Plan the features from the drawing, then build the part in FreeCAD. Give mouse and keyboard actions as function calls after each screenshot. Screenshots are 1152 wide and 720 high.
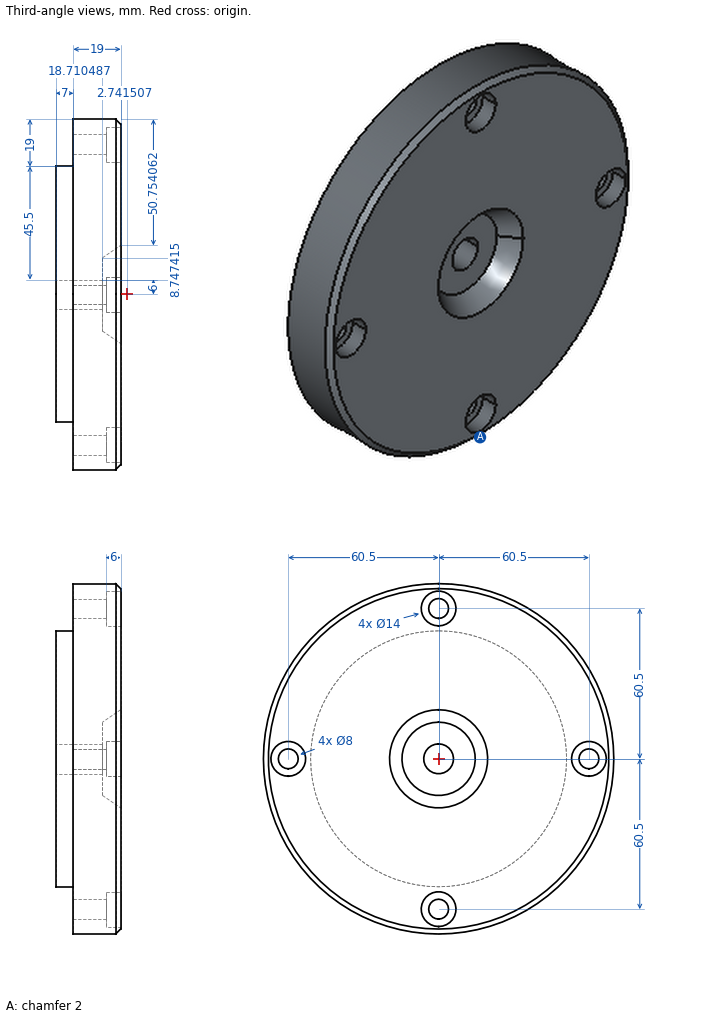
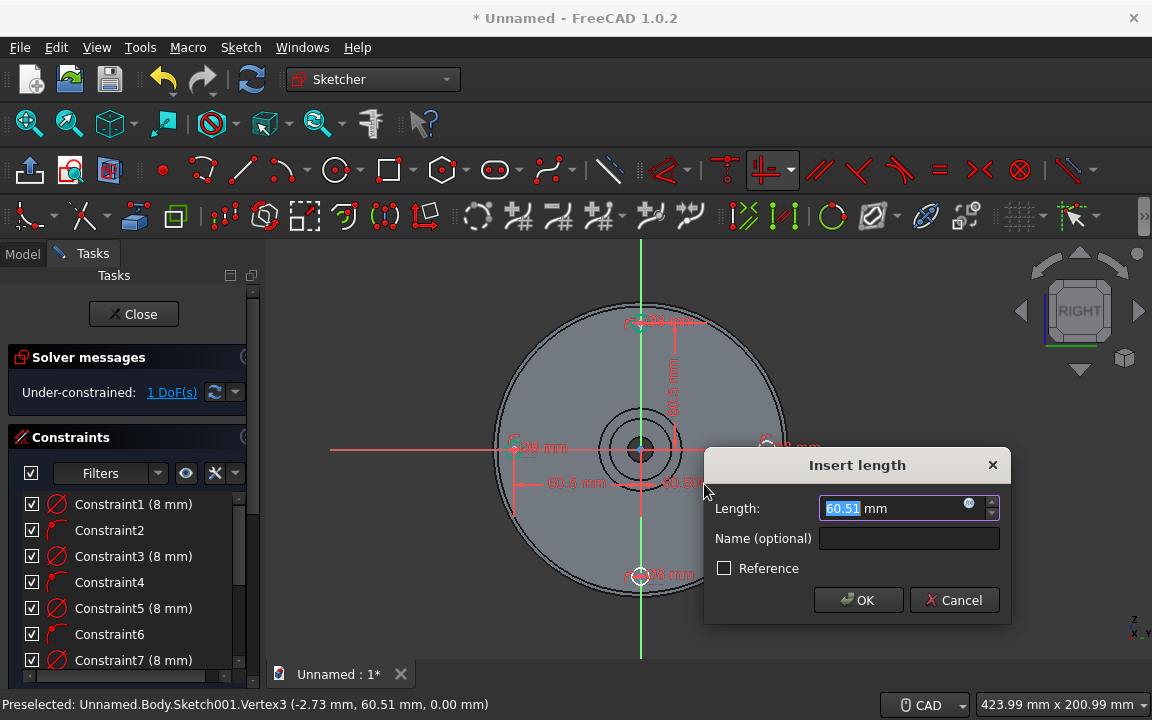
text(60.5)
key(Return)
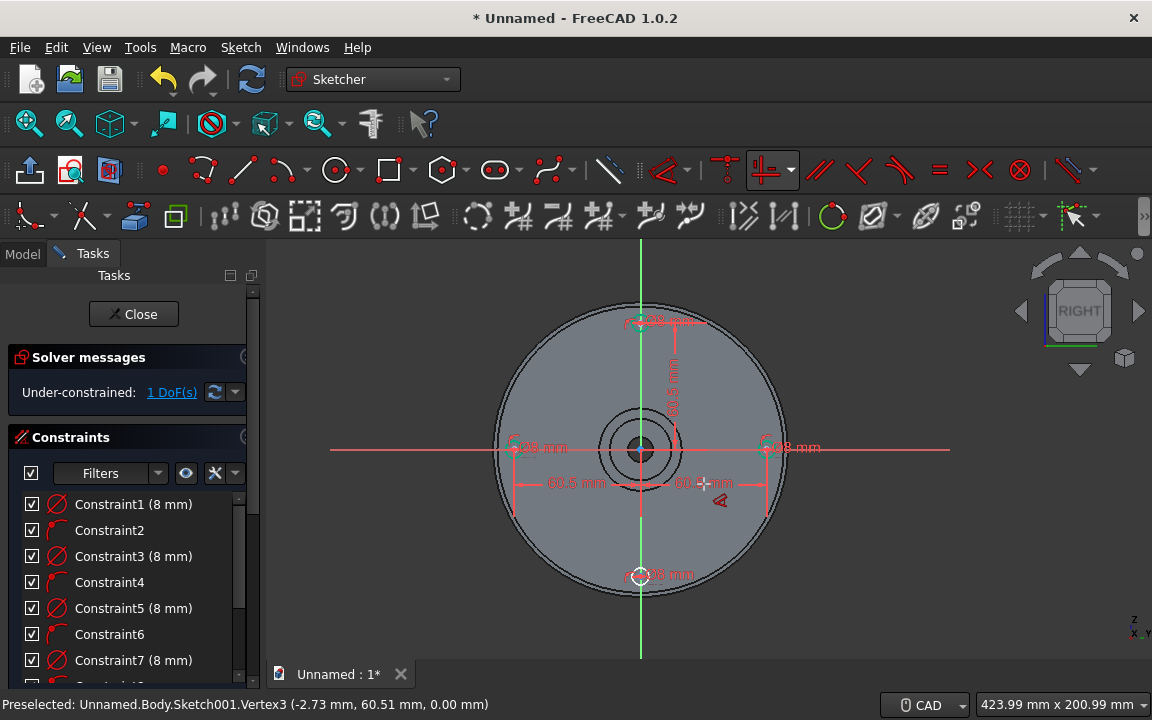
click(641, 577)
click(675, 513)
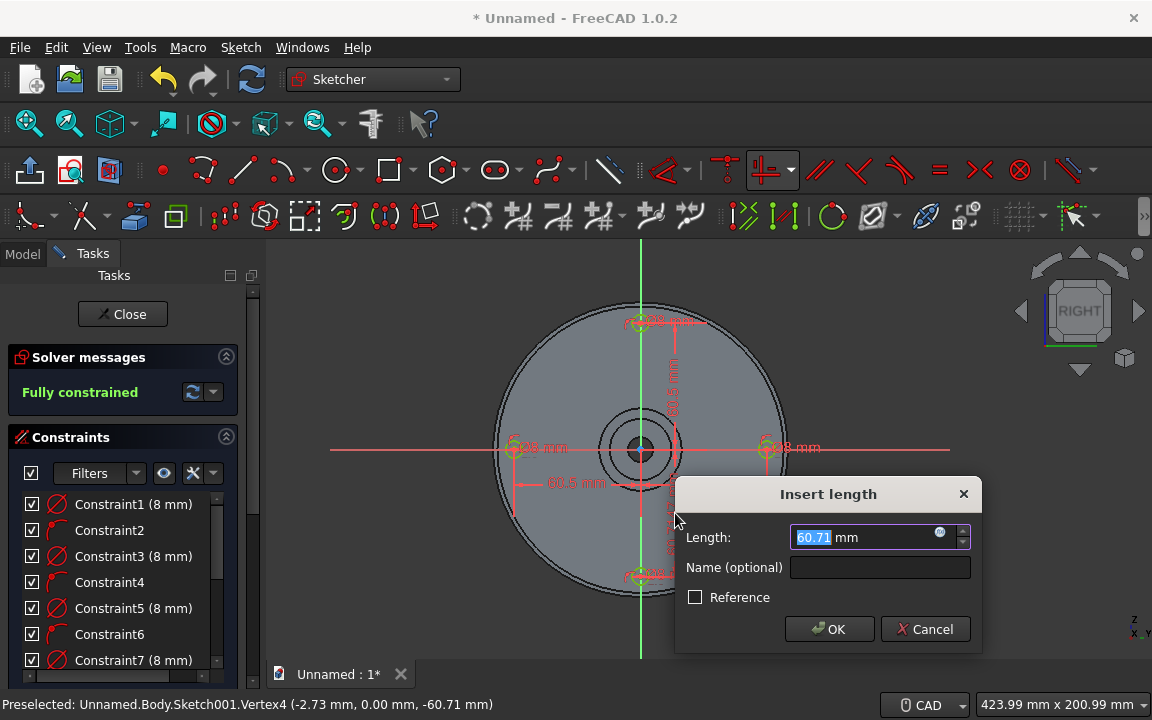
text(60.5)
key(Return)
key(Escape)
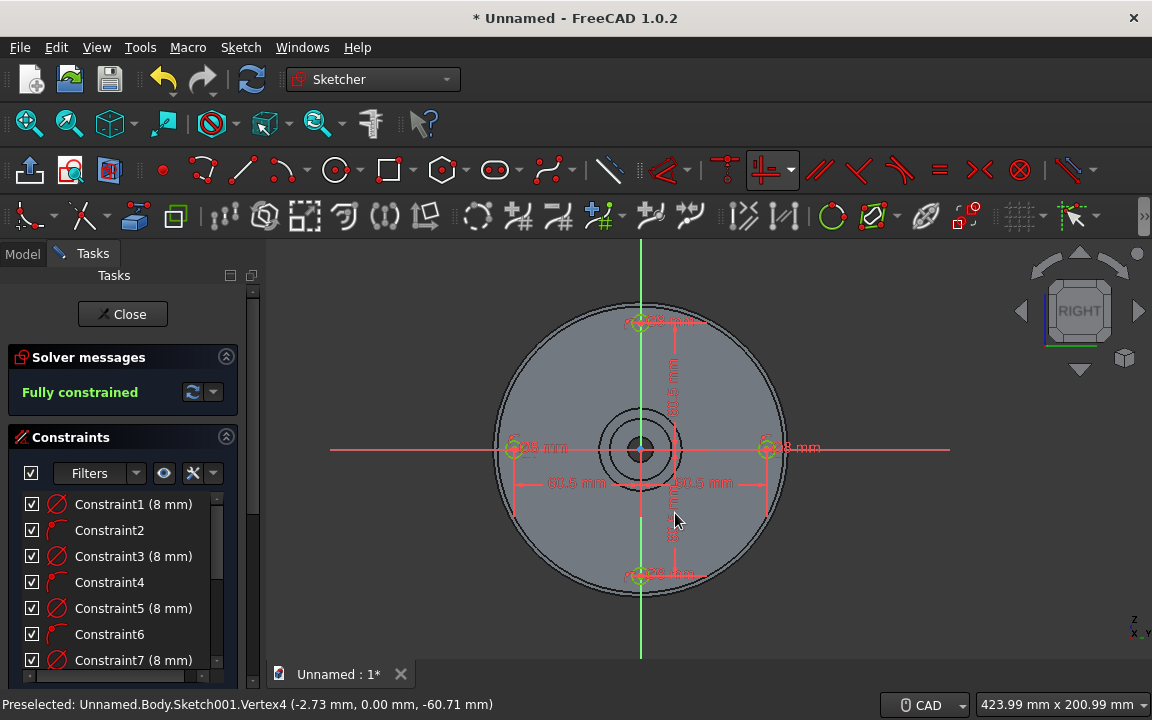
click(123, 314)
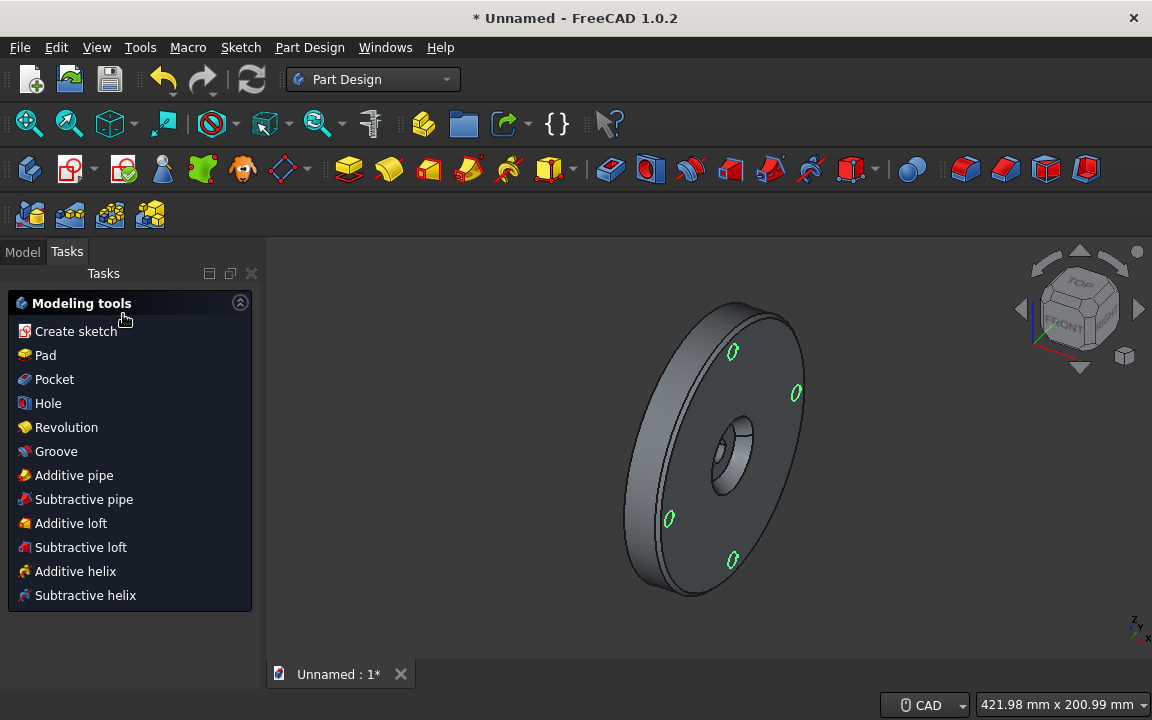
click(612, 170)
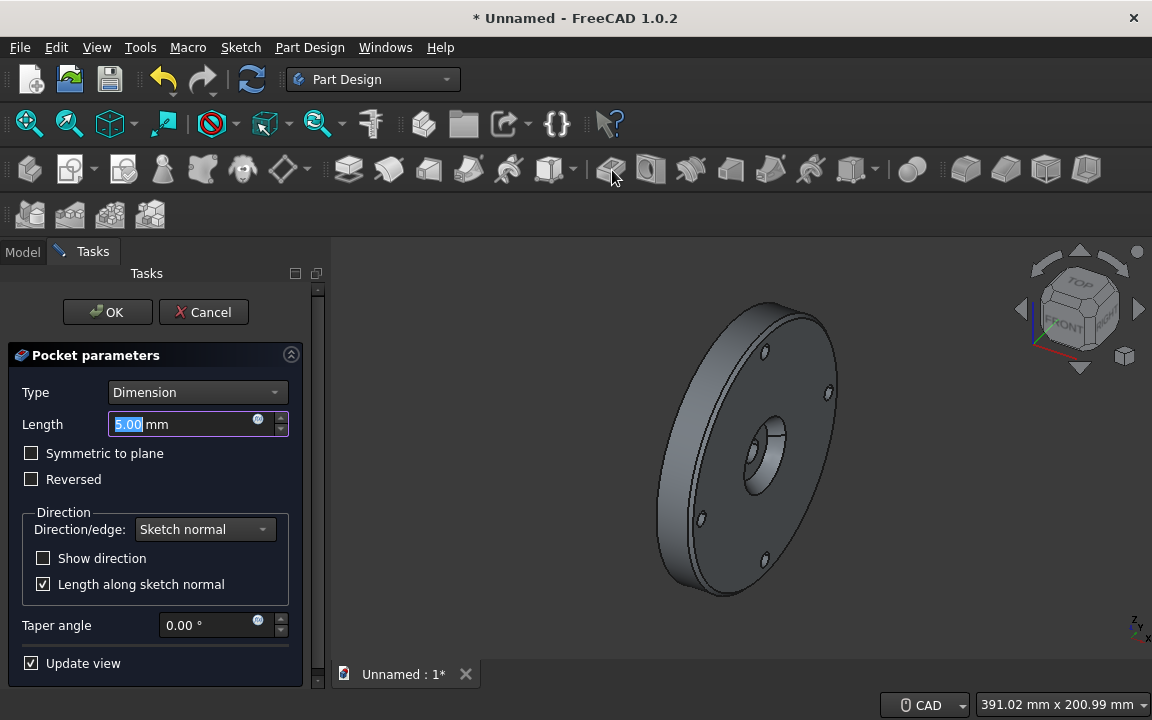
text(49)
key(Tab)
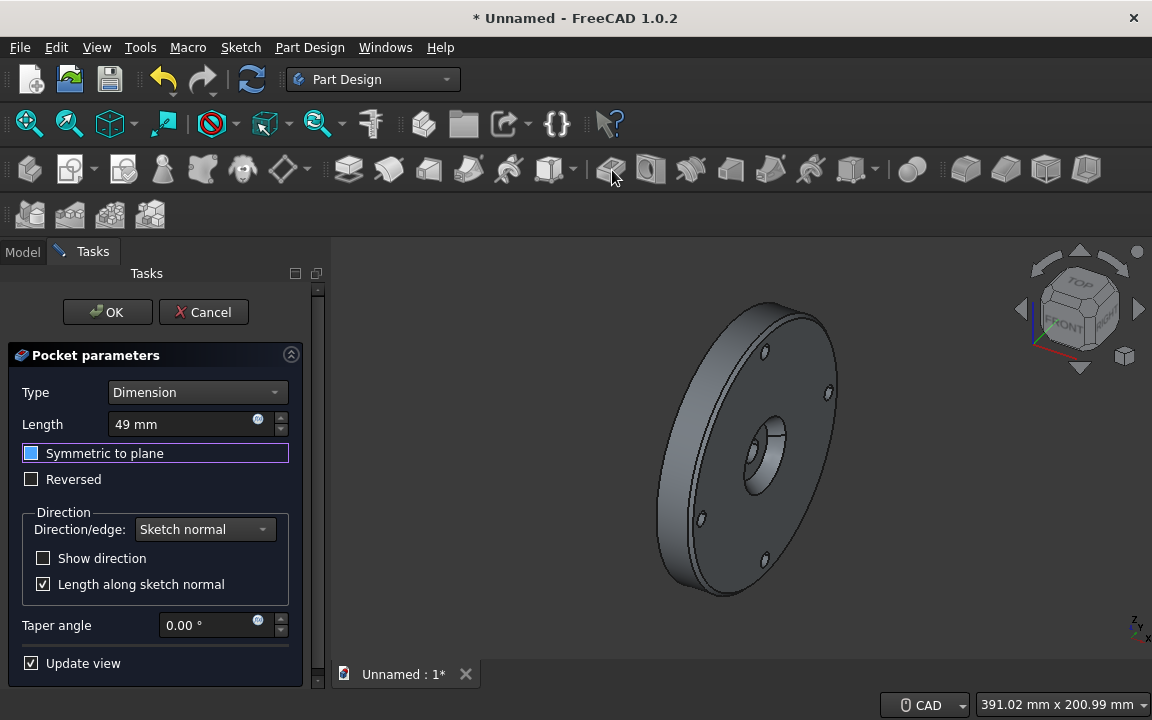
click(108, 312)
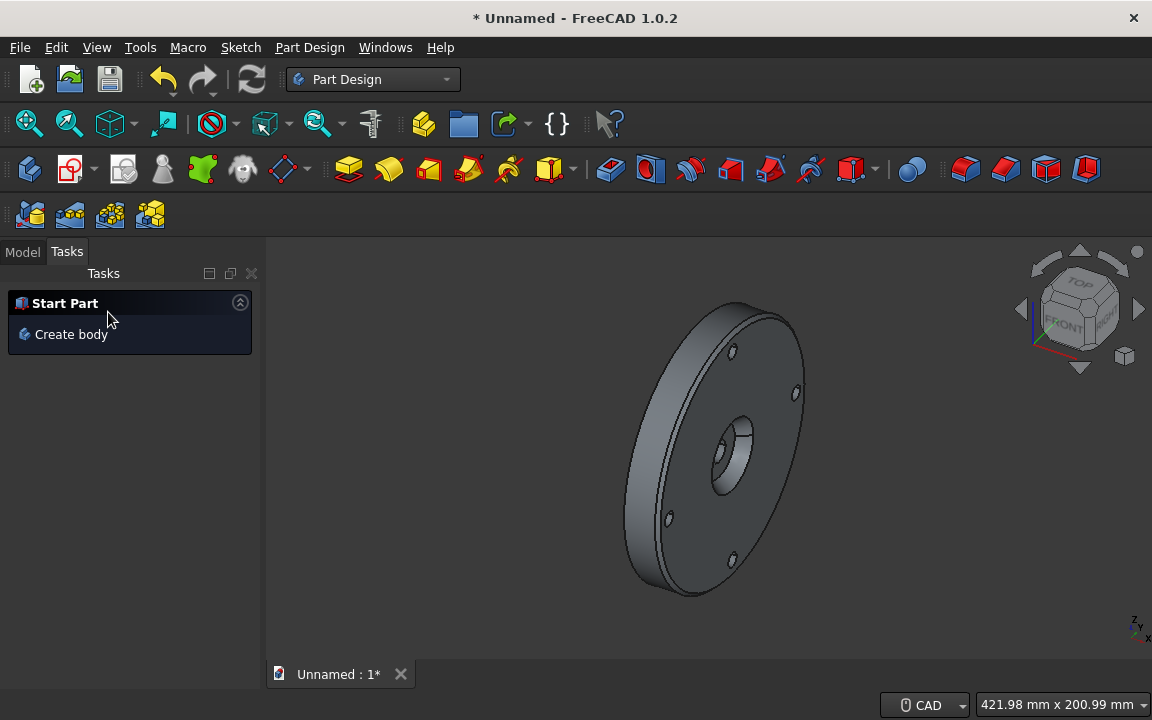
click(774, 380)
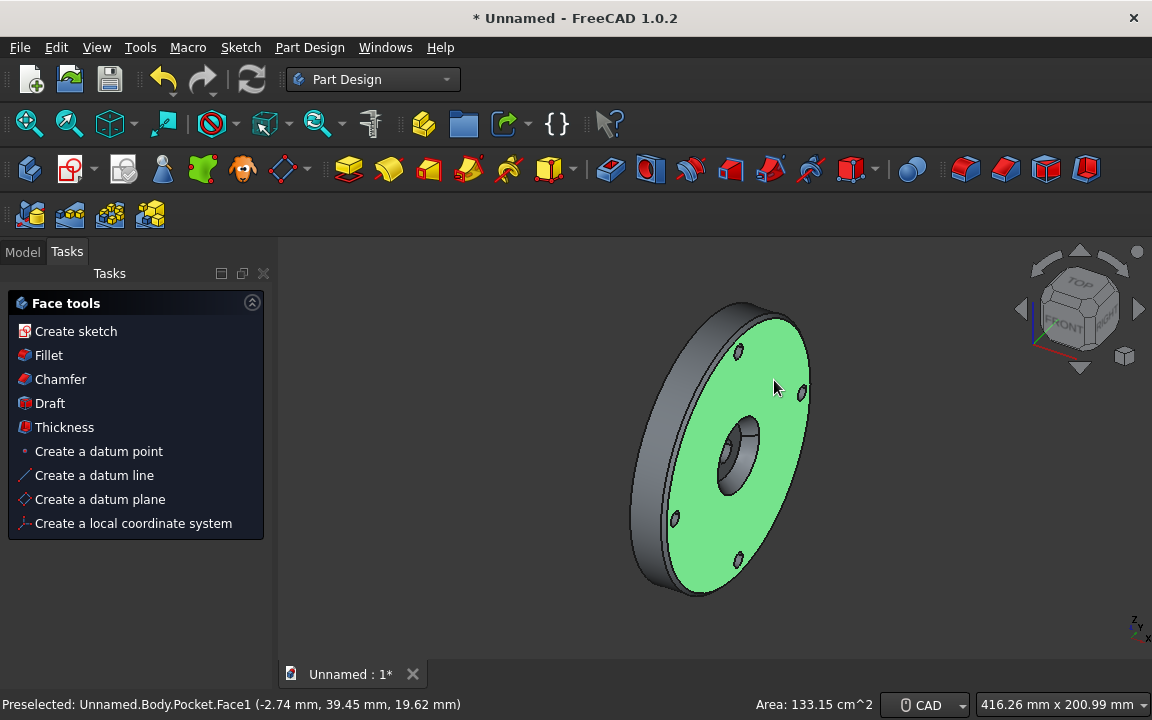
click(70, 170)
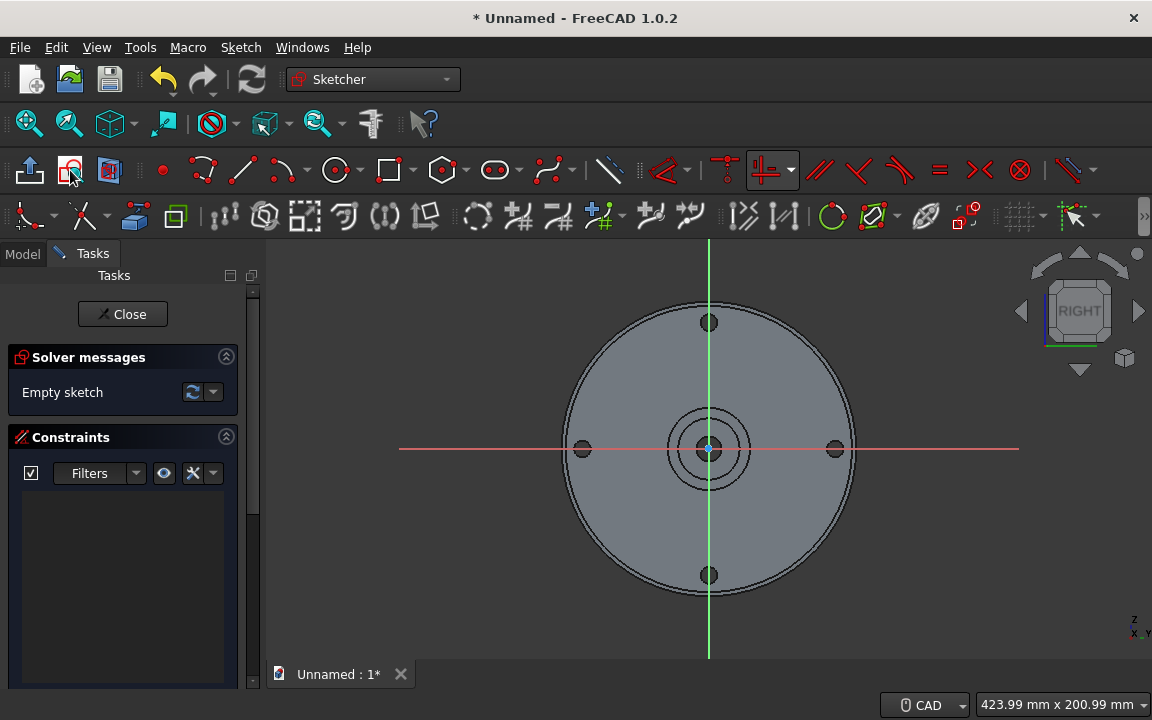
click(336, 170)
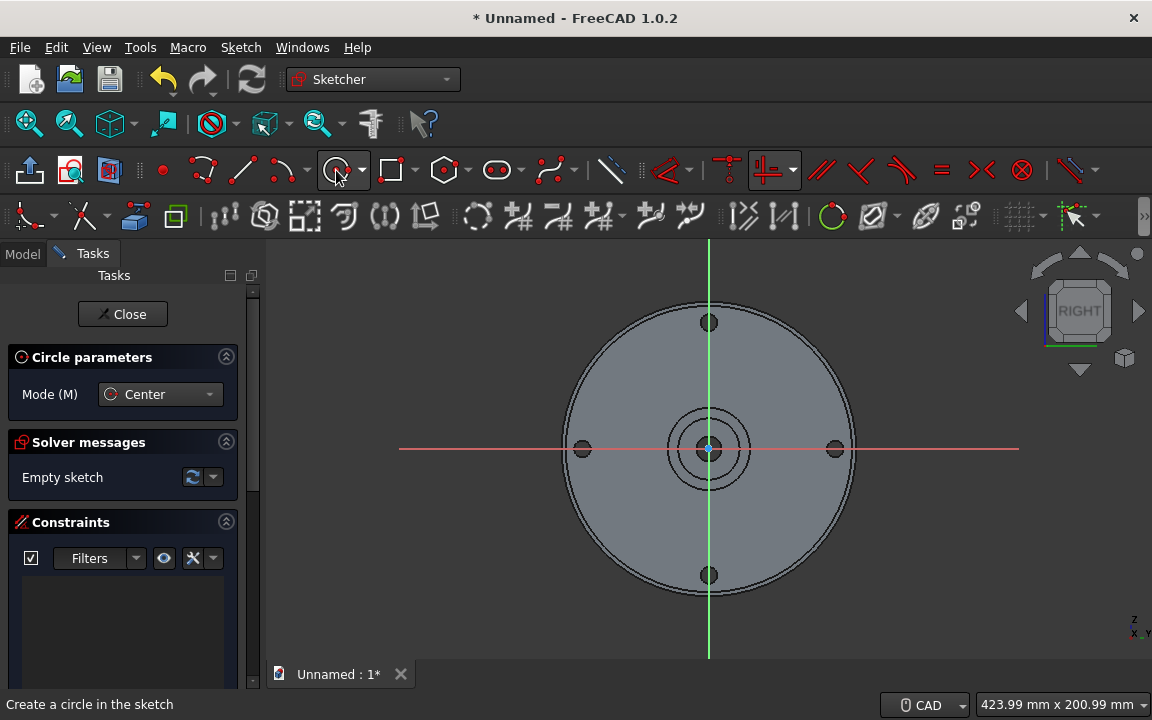
scroll(709, 323, up, 3)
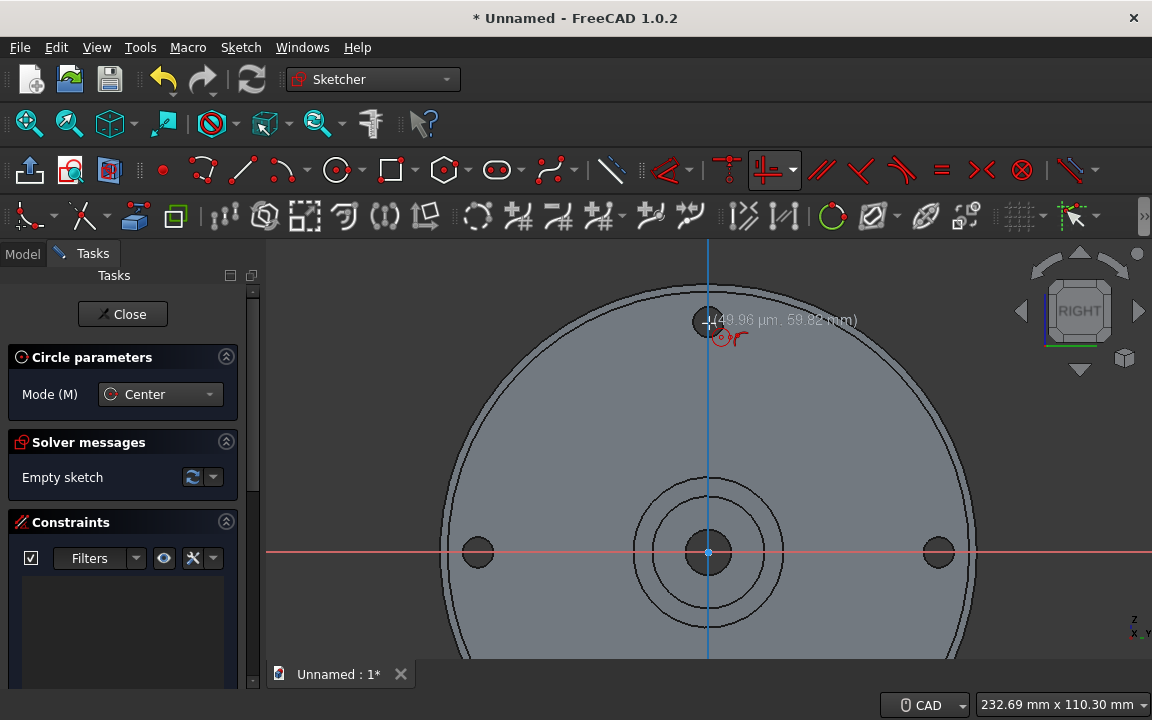
click(708, 322)
move(727, 303)